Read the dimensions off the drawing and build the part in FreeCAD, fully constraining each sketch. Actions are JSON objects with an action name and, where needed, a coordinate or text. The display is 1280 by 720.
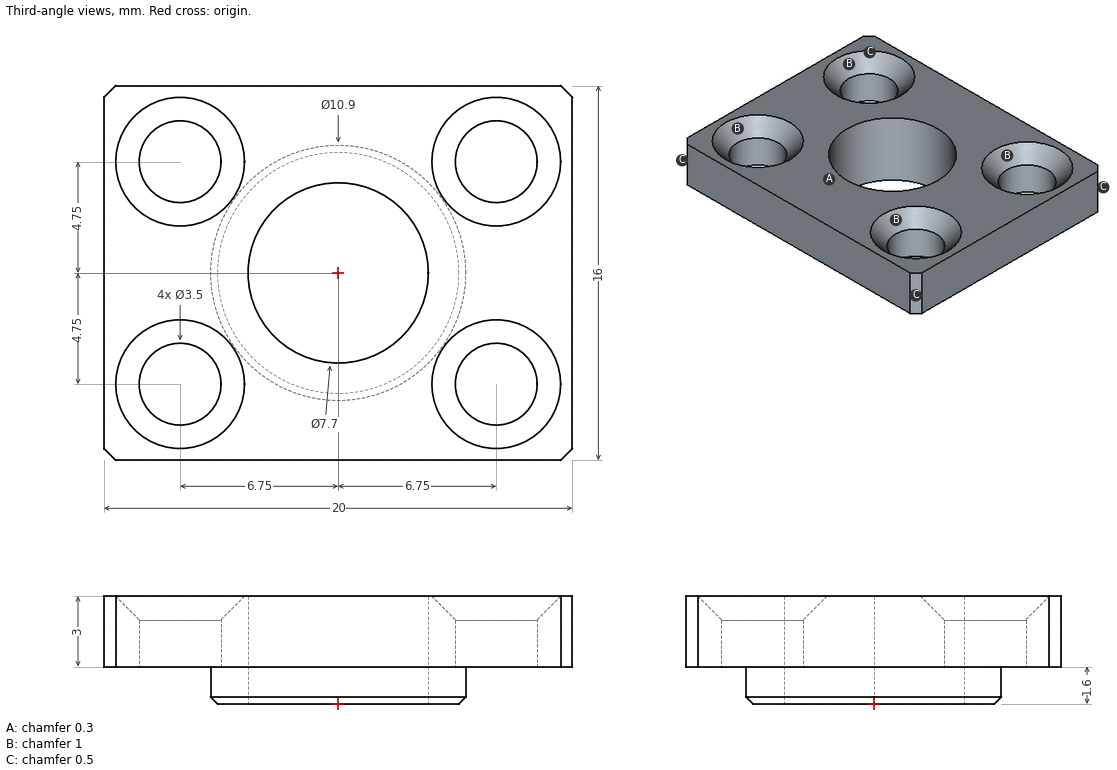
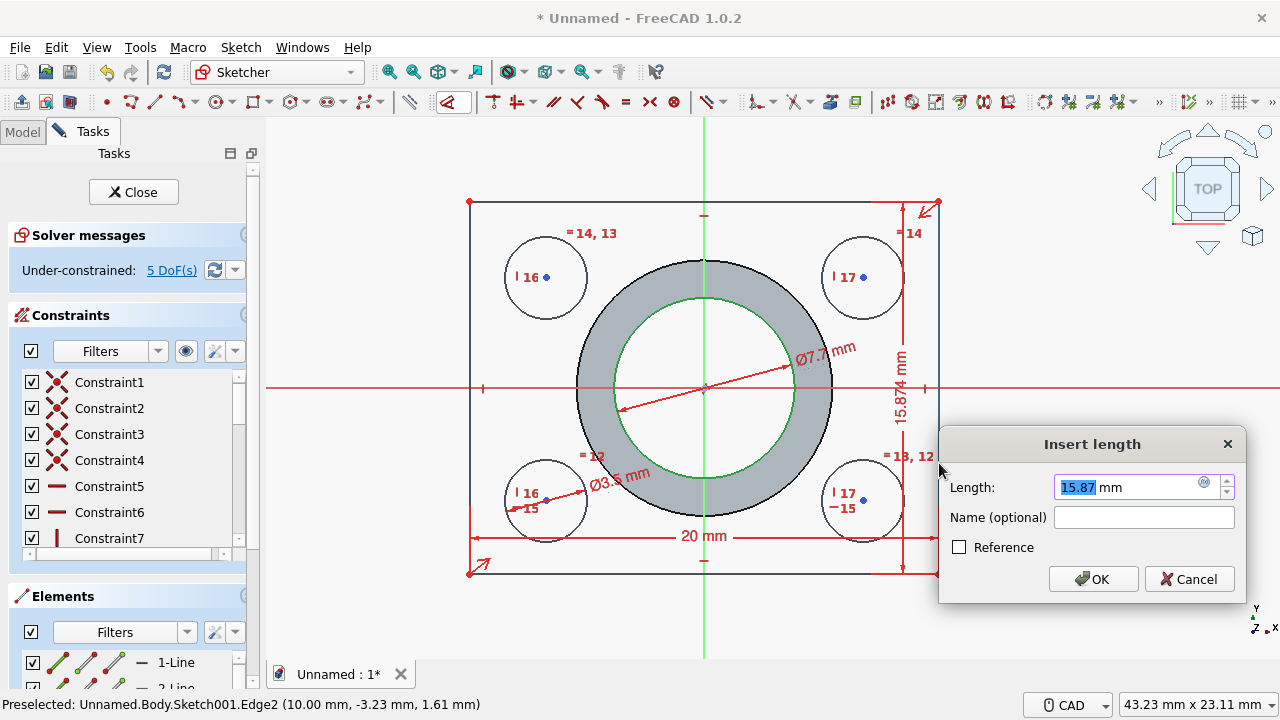
{"action": "type", "text": "16"}
{"action": "key", "text": "Return"}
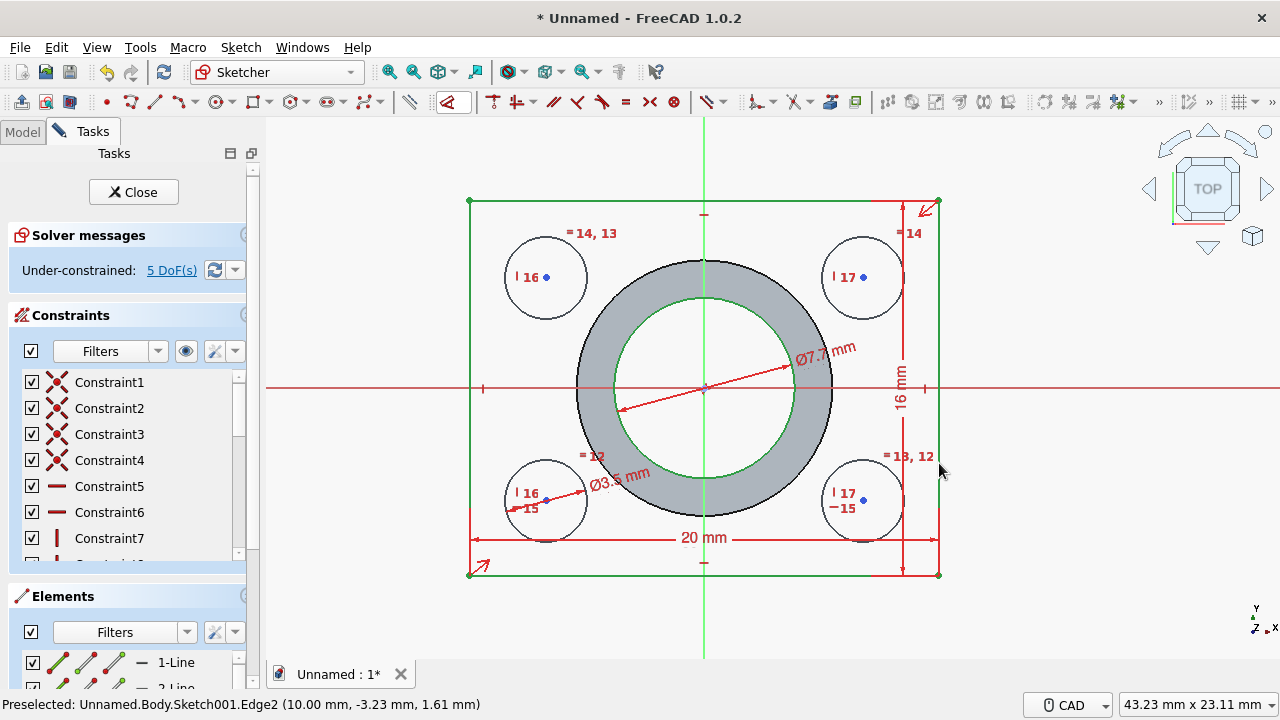
{"action": "left_click", "coordinate": [546, 501]}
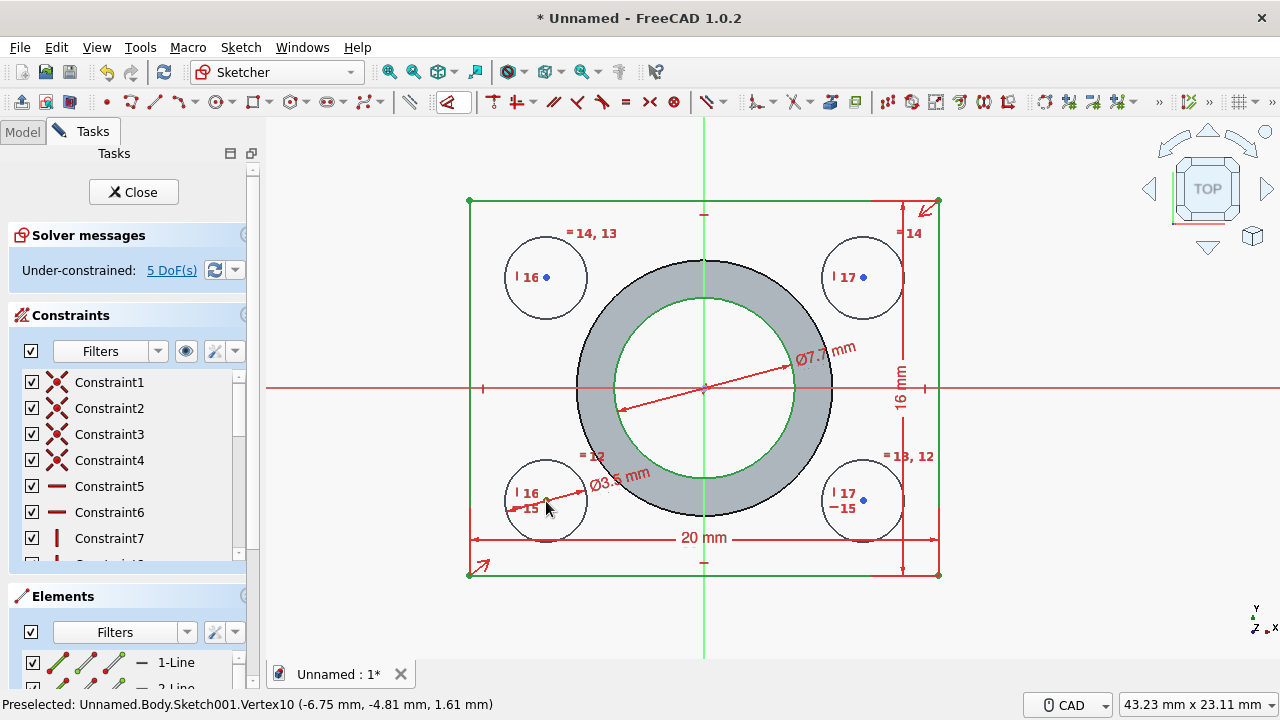
{"action": "left_click", "coordinate": [466, 102]}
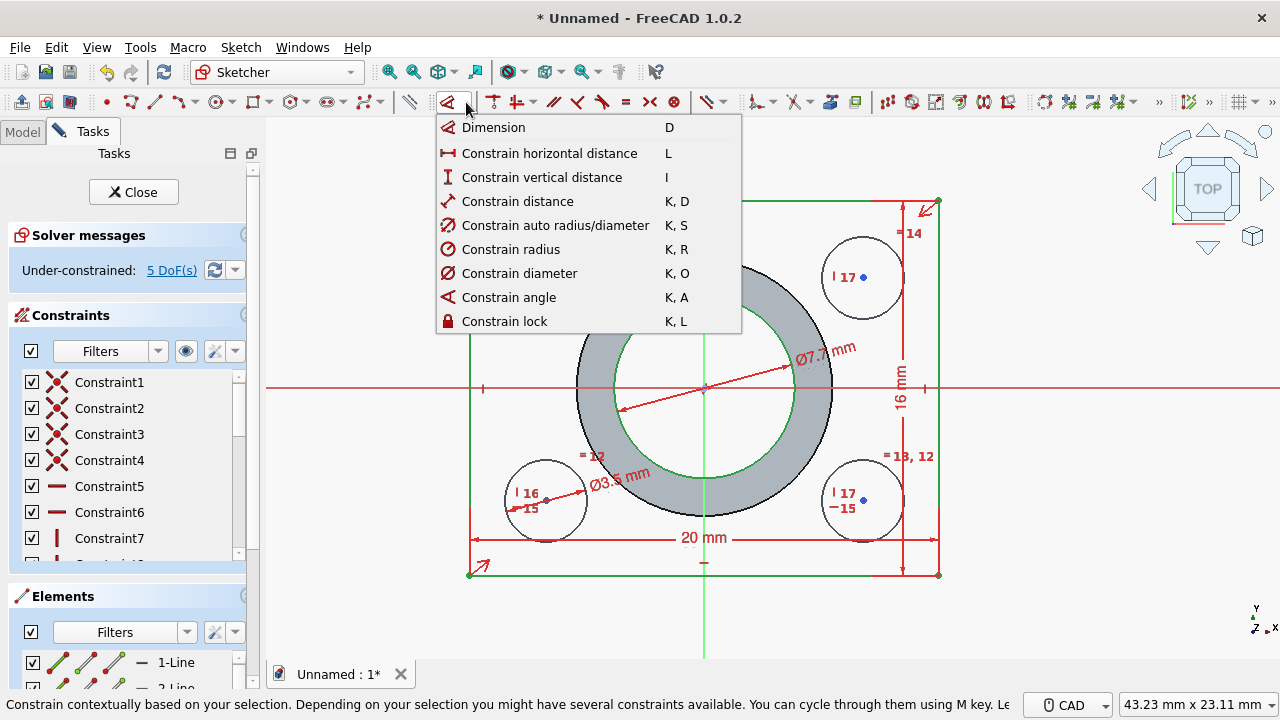
{"action": "left_click", "coordinate": [589, 153]}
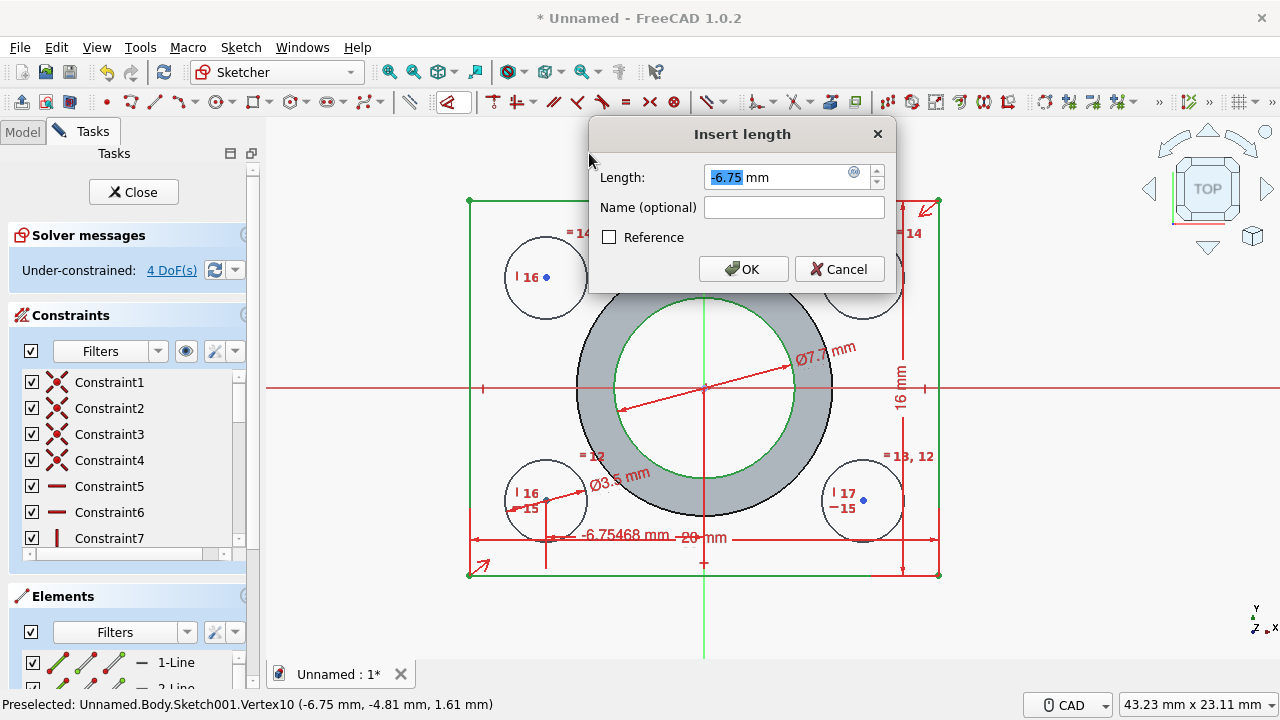
{"action": "type", "text": "-6.75"}
{"action": "key", "text": "Return"}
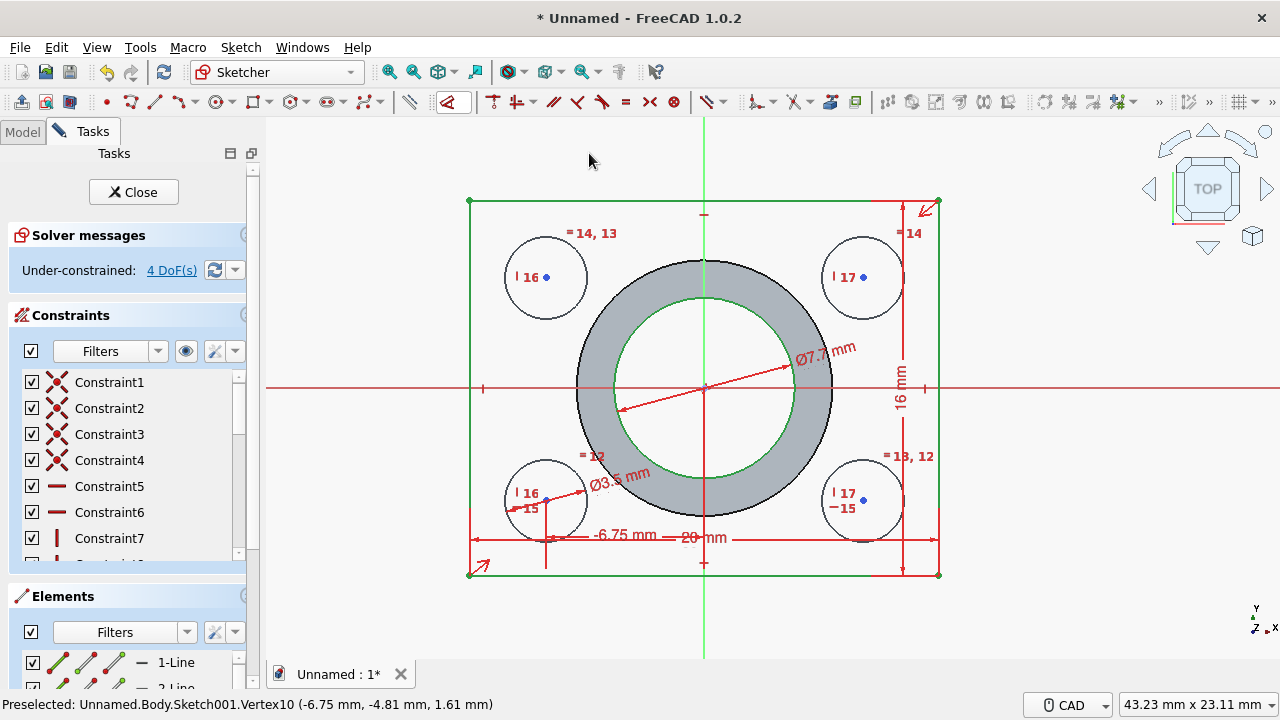
{"action": "left_click", "coordinate": [546, 501]}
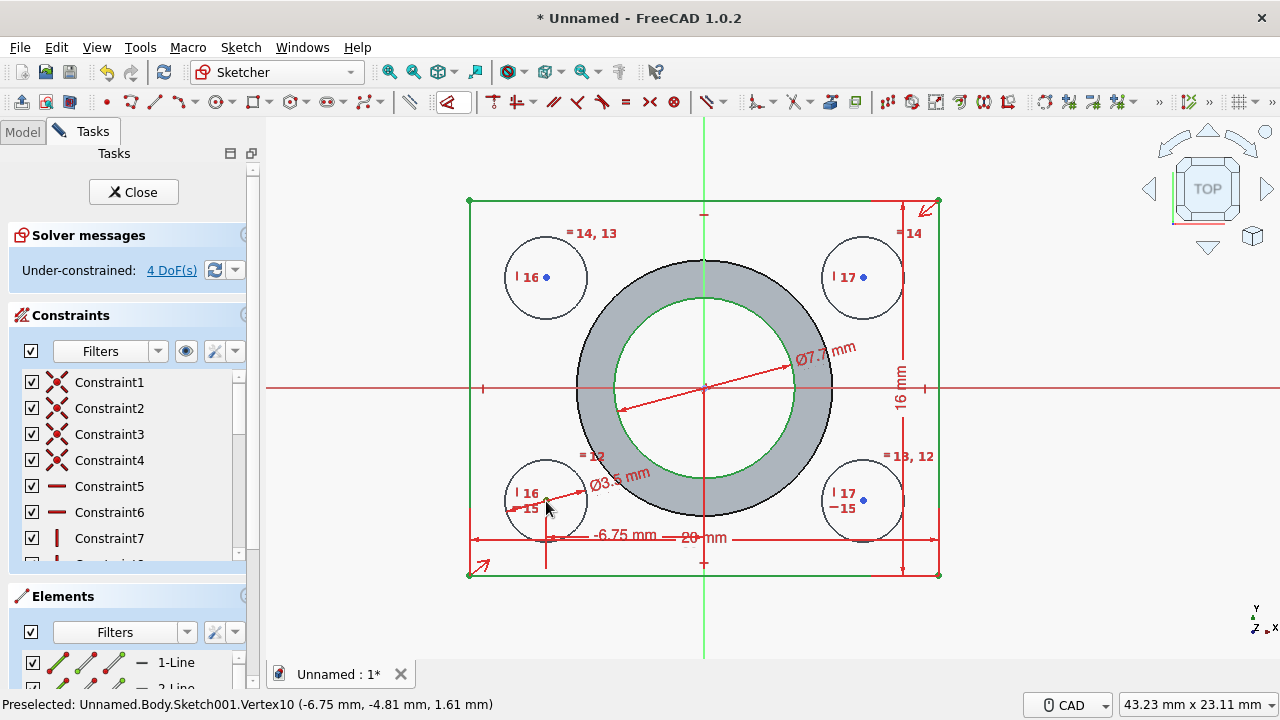
{"action": "key", "text": "i"}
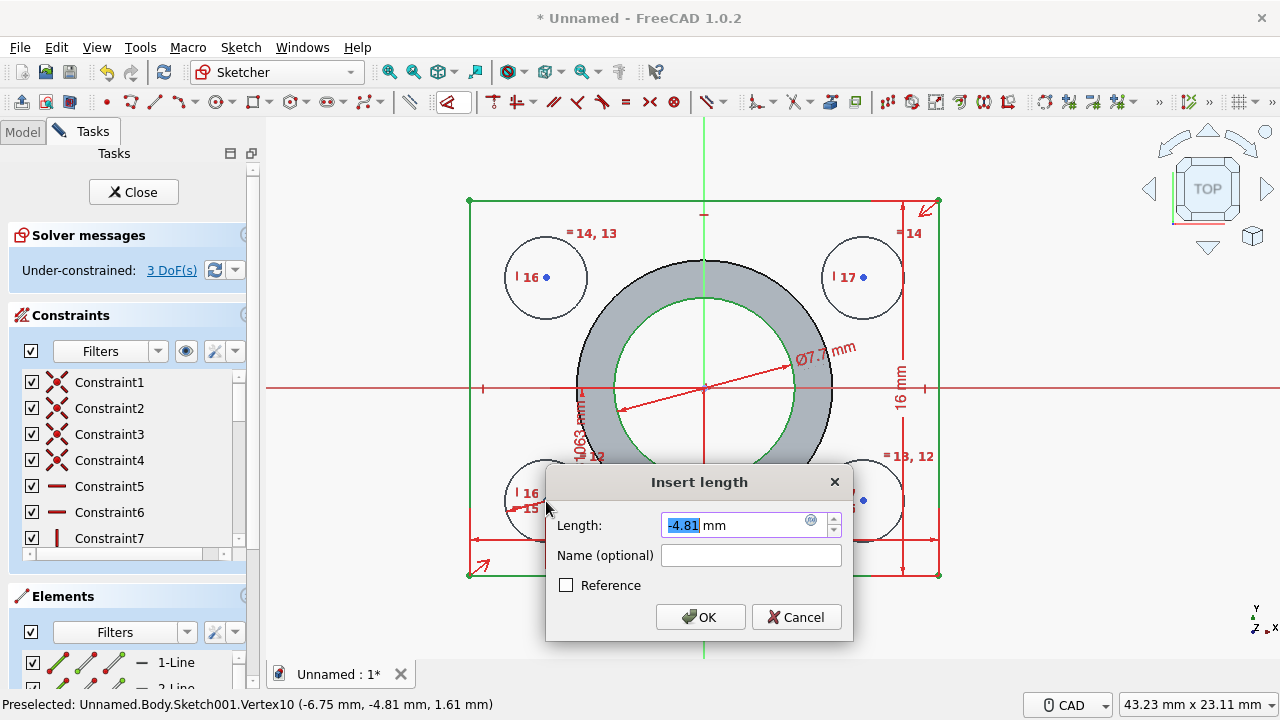
{"action": "type", "text": "-4.75"}
{"action": "key", "text": "Return"}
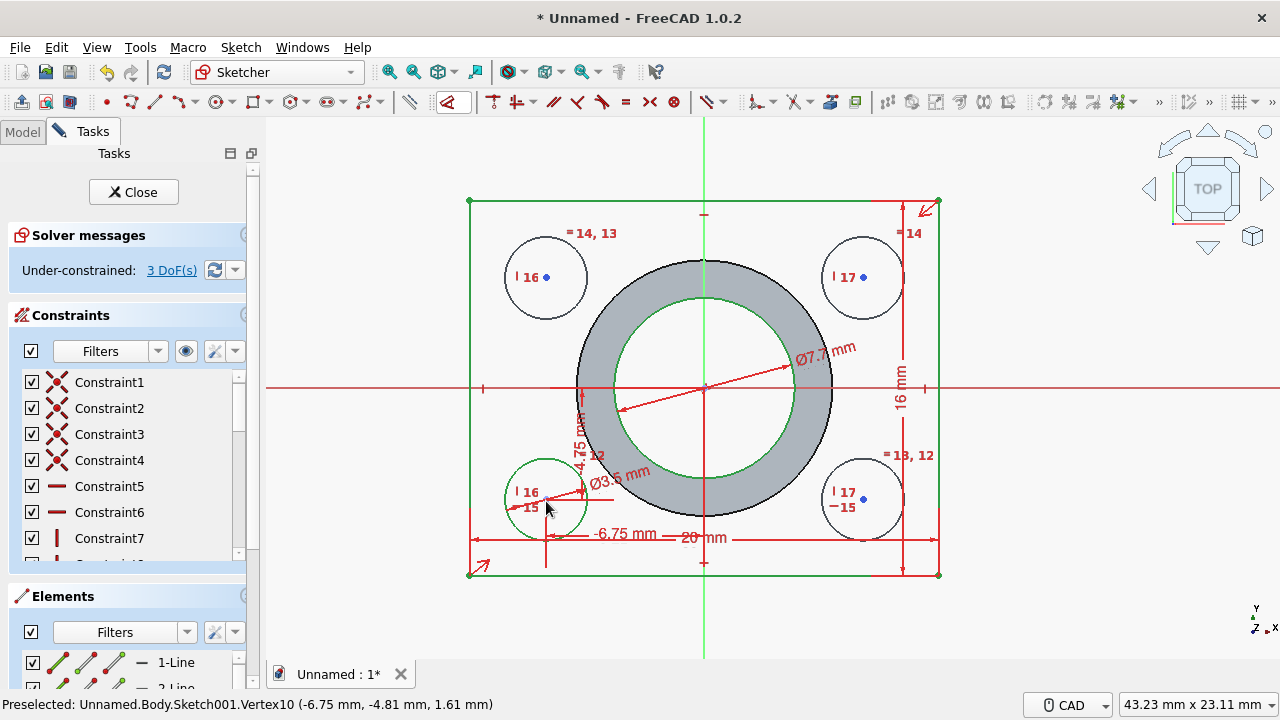
{"action": "left_click", "coordinate": [863, 500]}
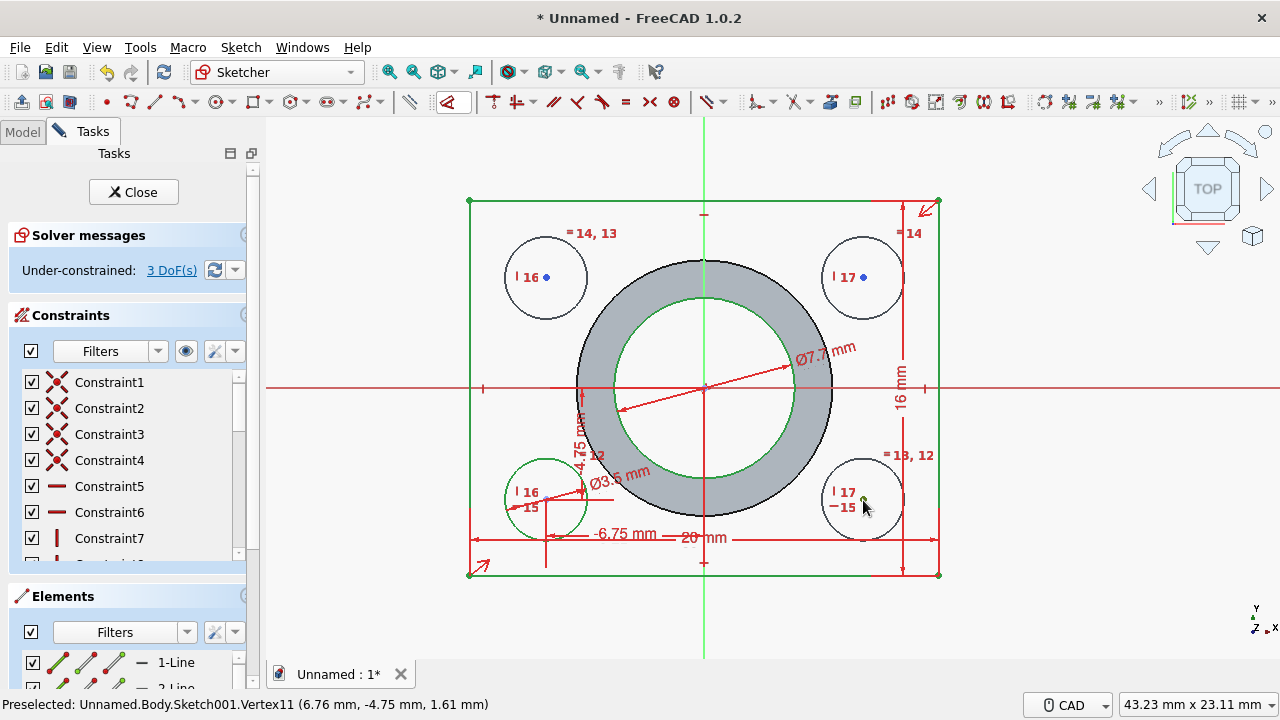
{"action": "key", "text": "l"}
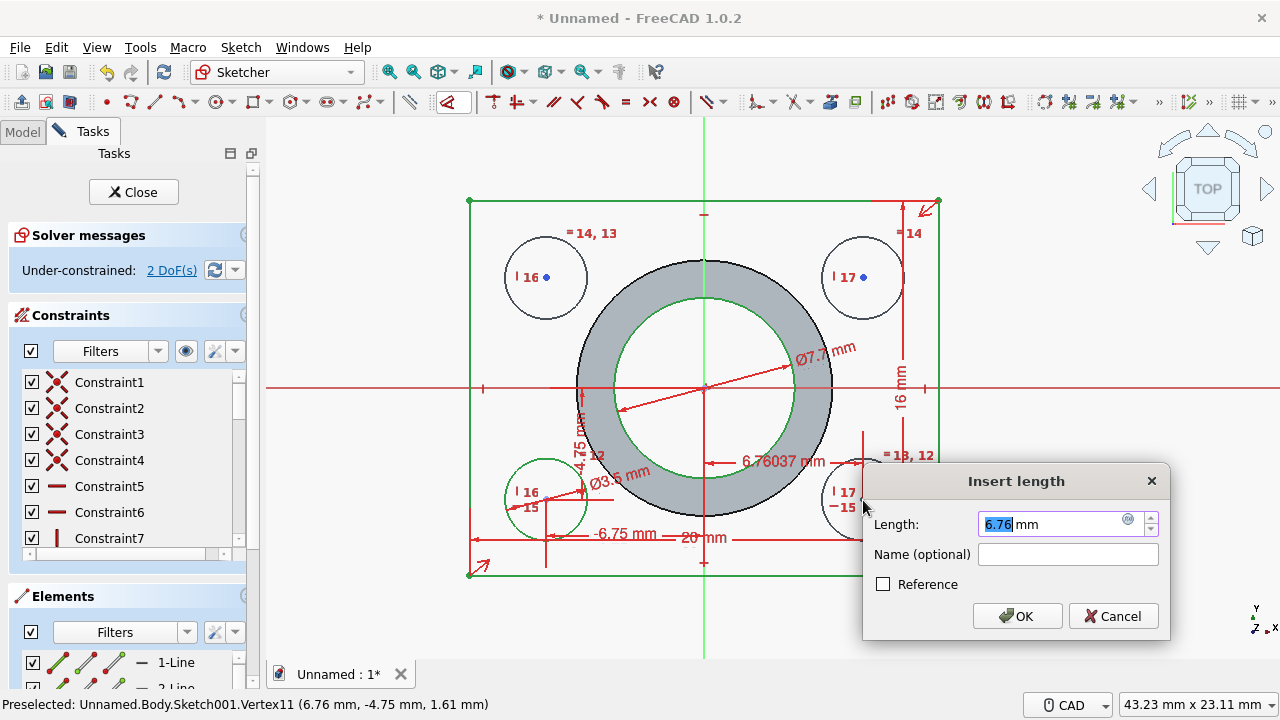
{"action": "type", "text": "6.75"}
{"action": "key", "text": "Return"}